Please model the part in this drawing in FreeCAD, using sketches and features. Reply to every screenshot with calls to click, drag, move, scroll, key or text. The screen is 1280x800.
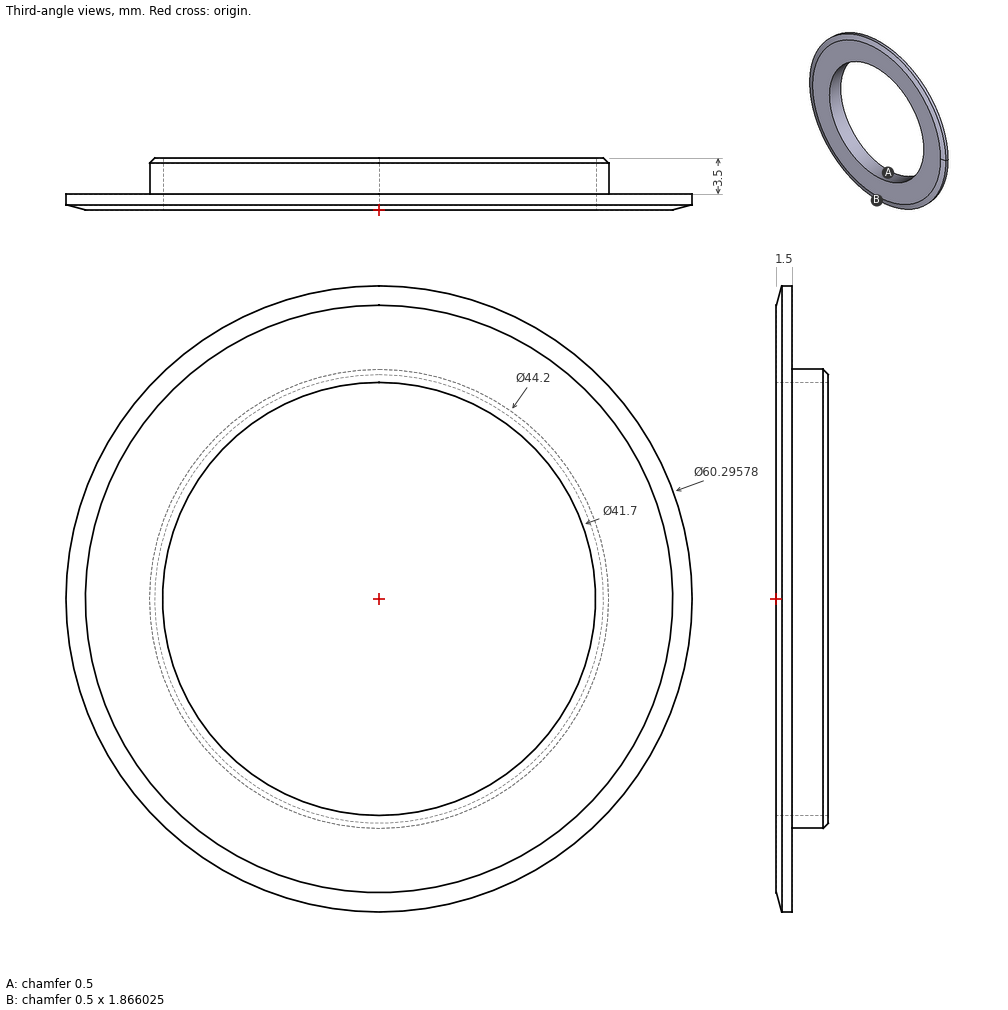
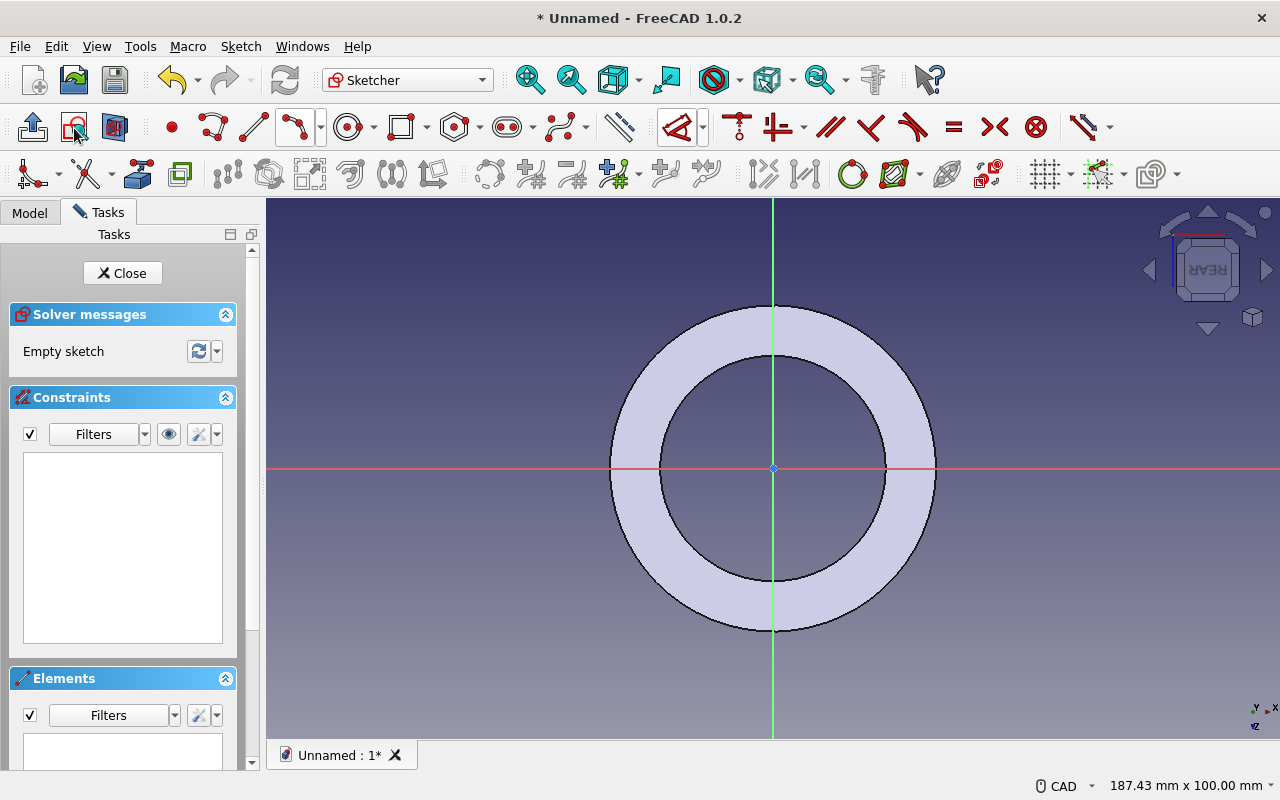
scroll(912, 469, up, 2)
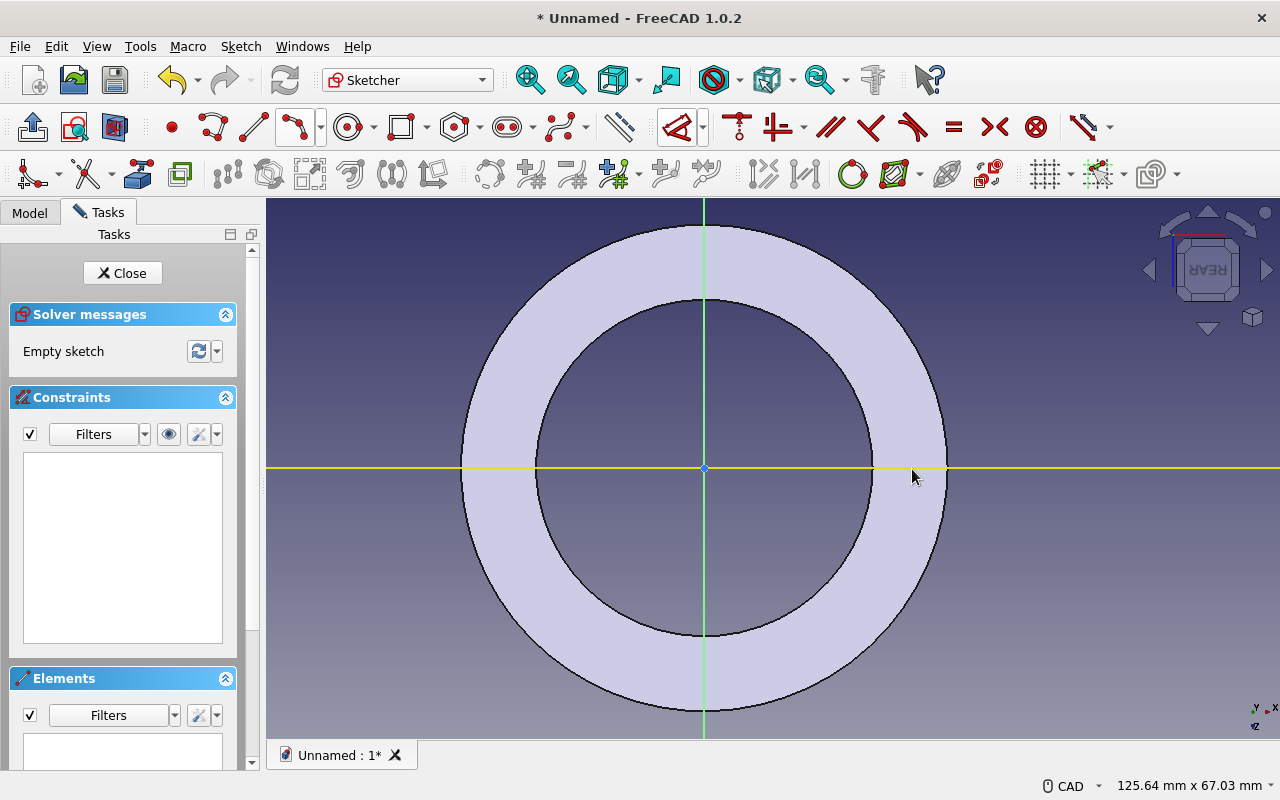
click(348, 128)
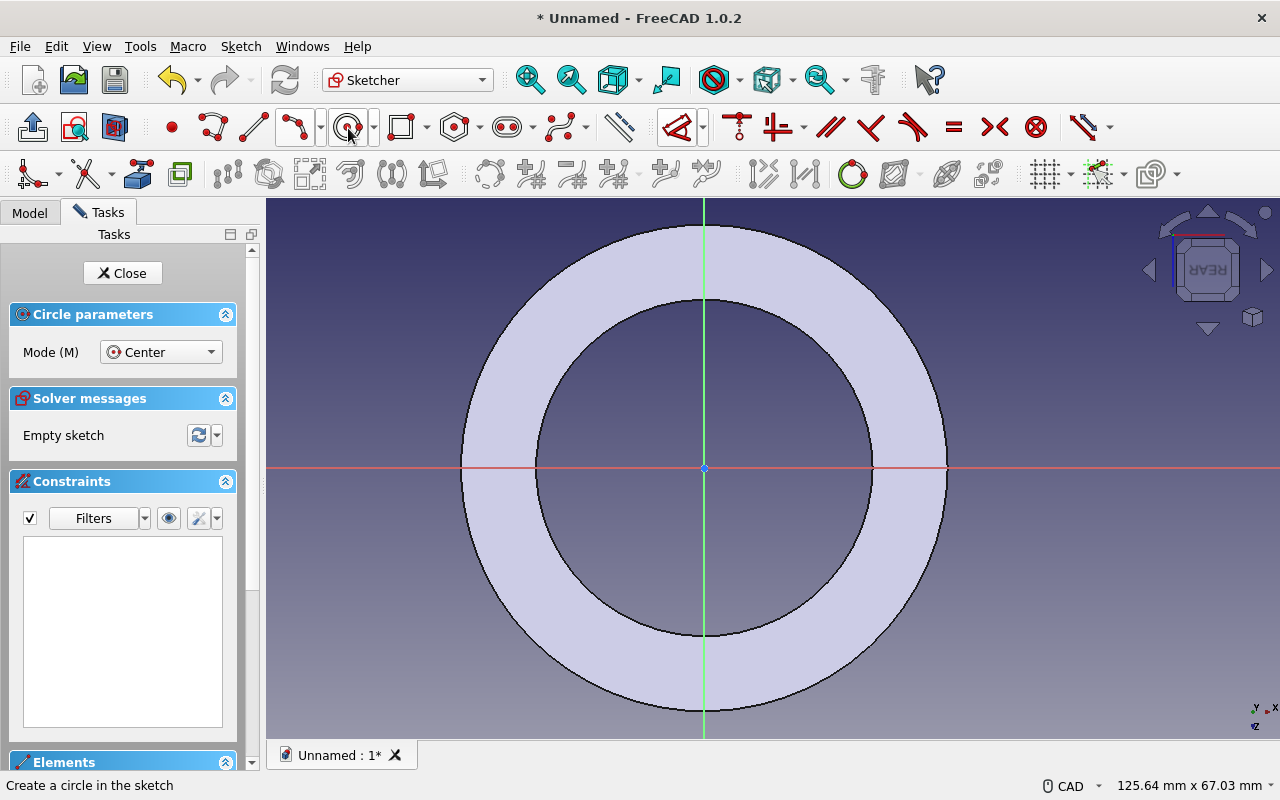
click(704, 468)
click(830, 342)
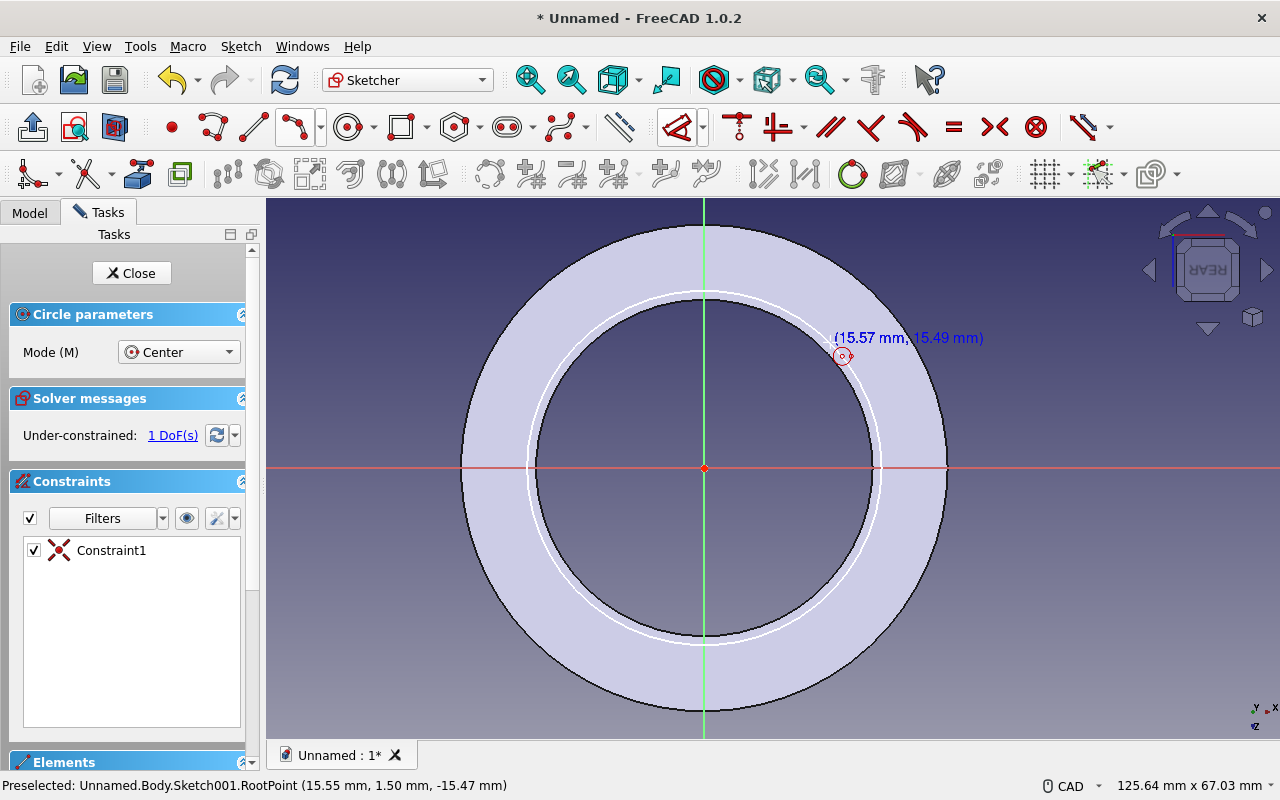
click(704, 468)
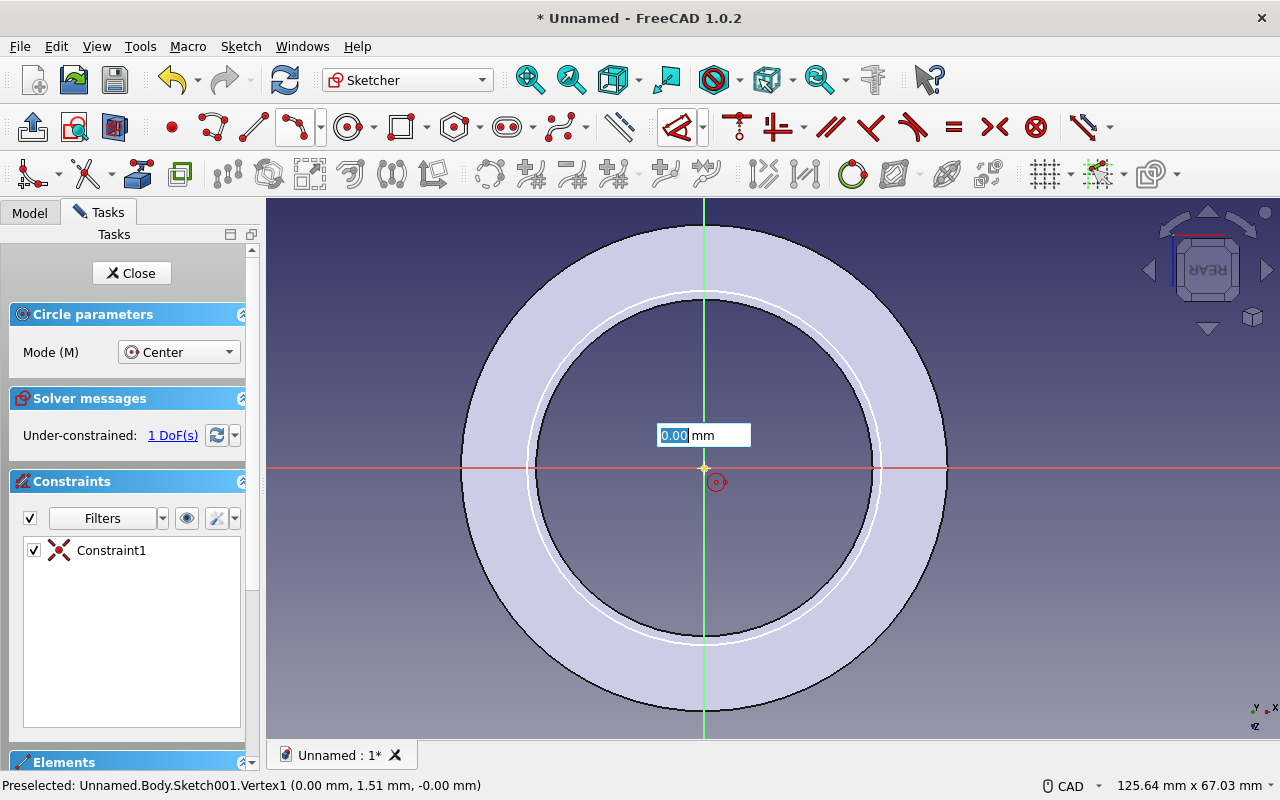
scroll(823, 349, up, 3)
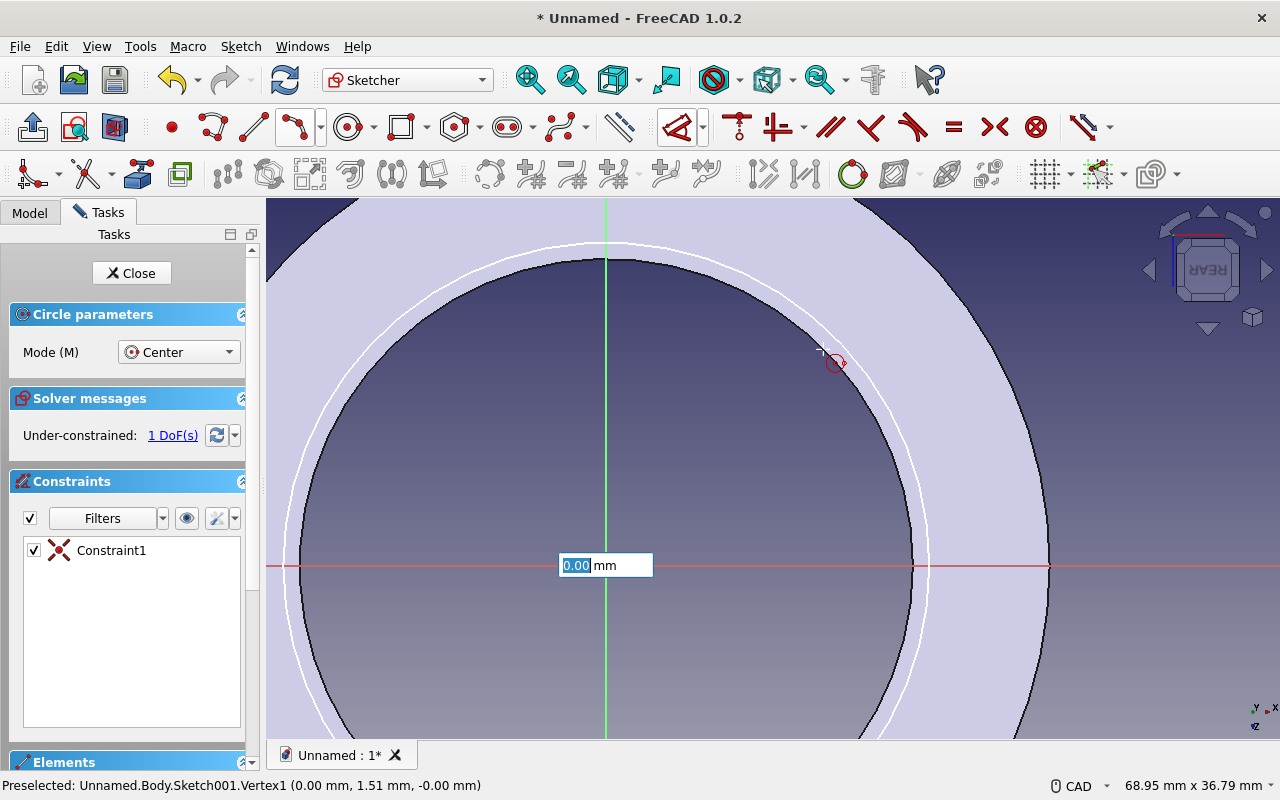
click(823, 349)
key(Escape)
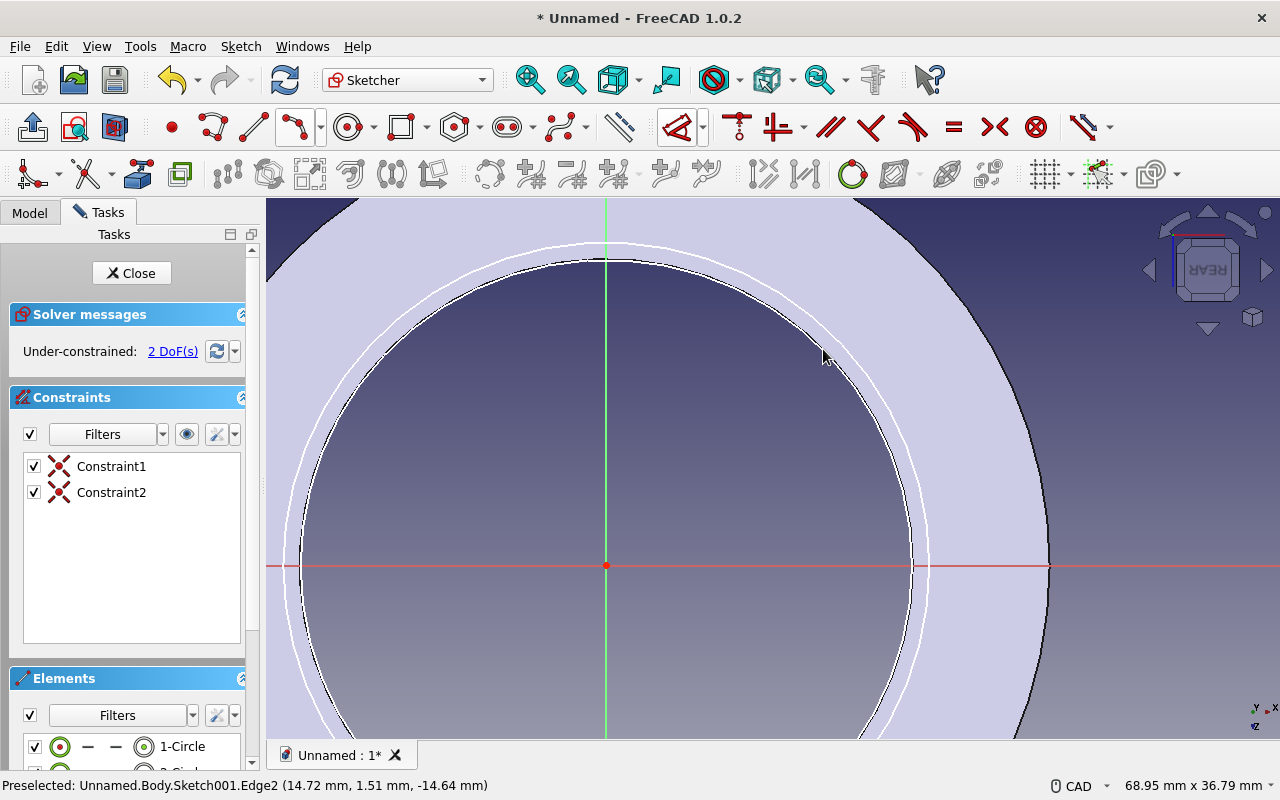
click(676, 128)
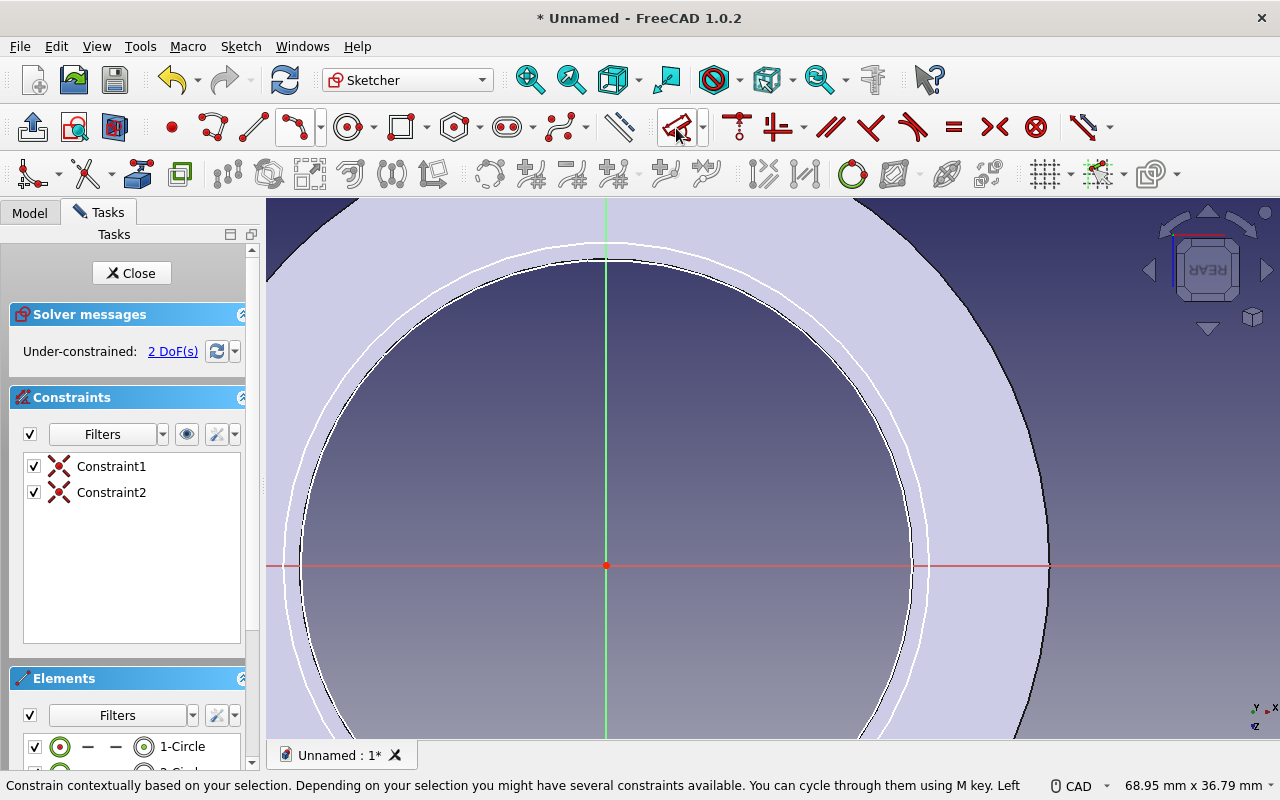
click(834, 337)
click(857, 314)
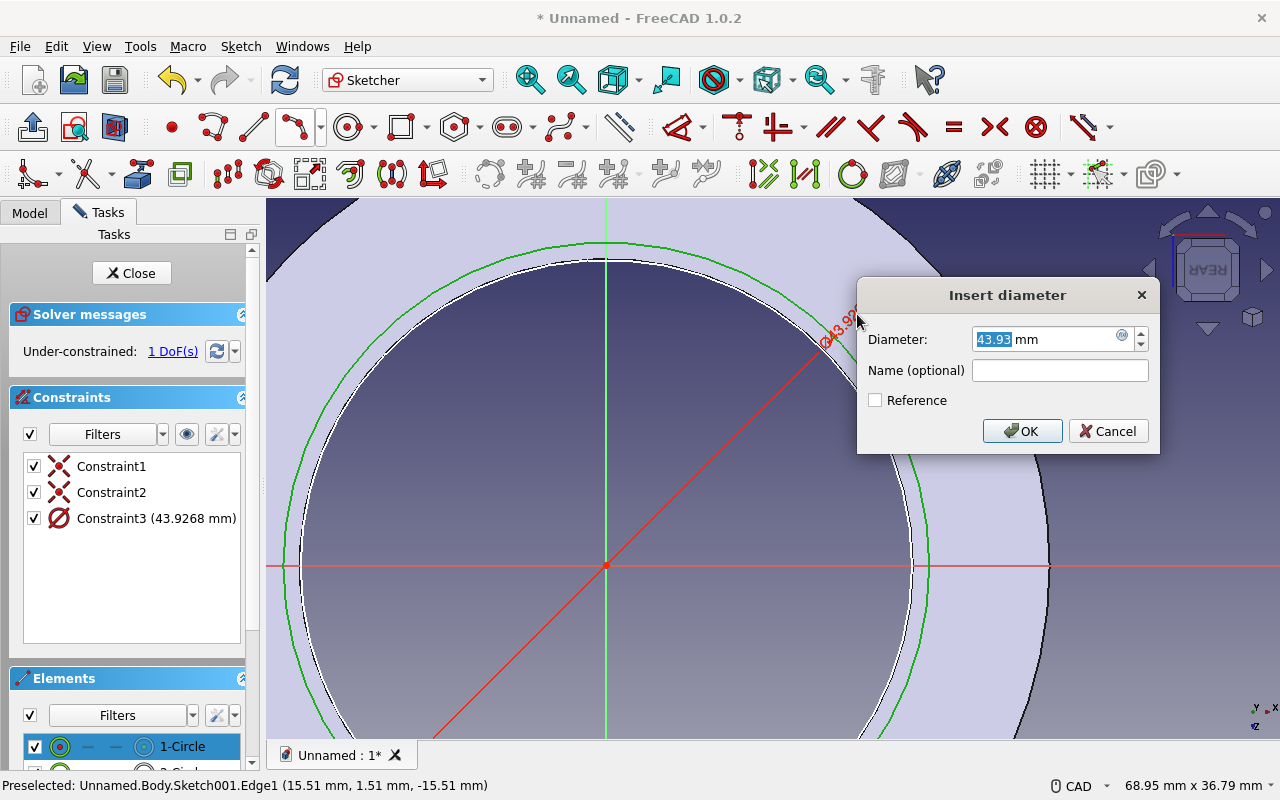
text(44.2)
key(Return)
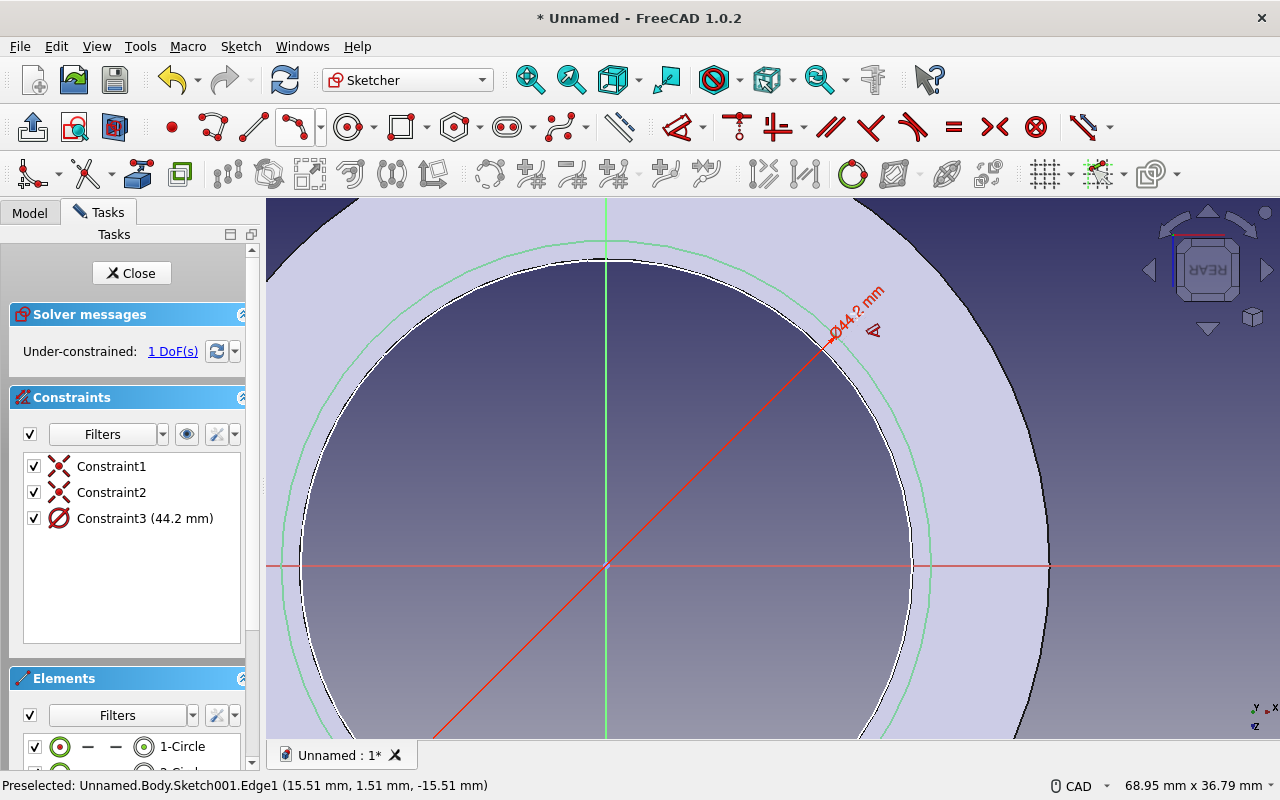
click(822, 349)
click(952, 463)